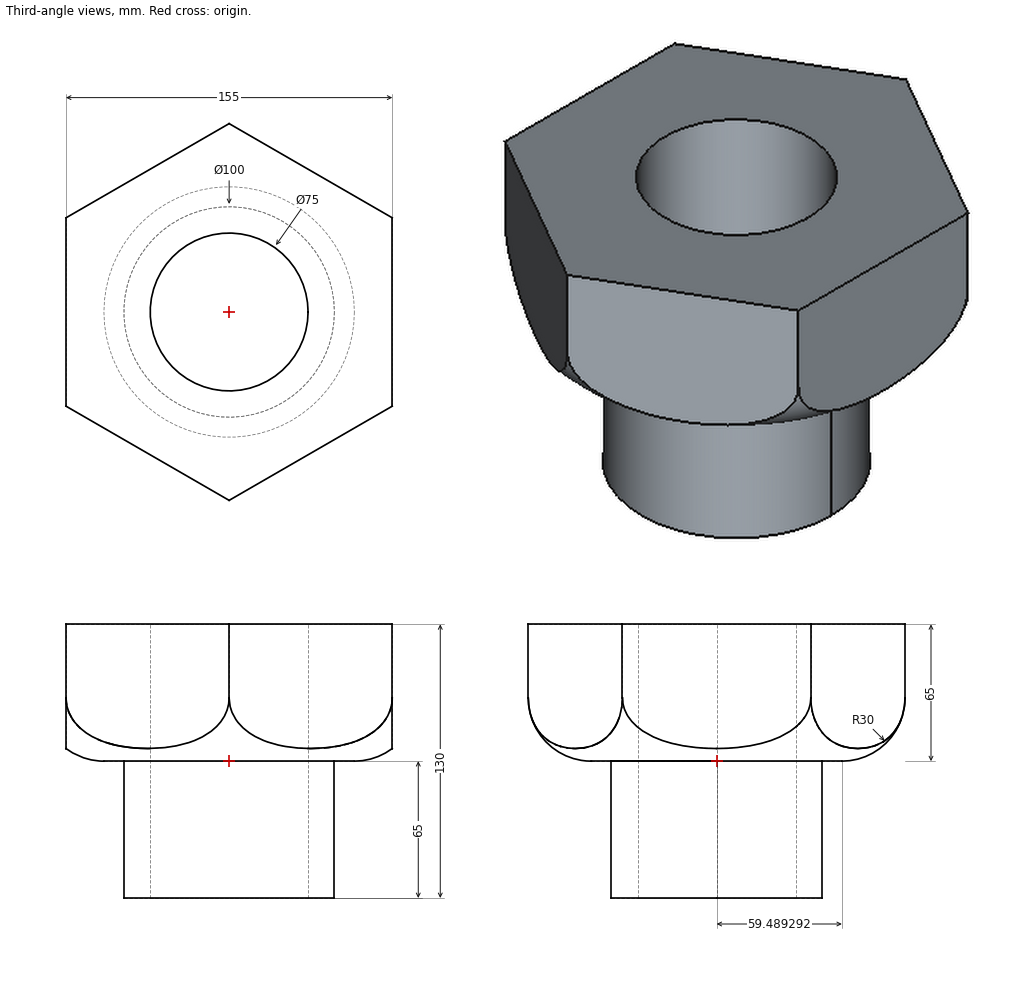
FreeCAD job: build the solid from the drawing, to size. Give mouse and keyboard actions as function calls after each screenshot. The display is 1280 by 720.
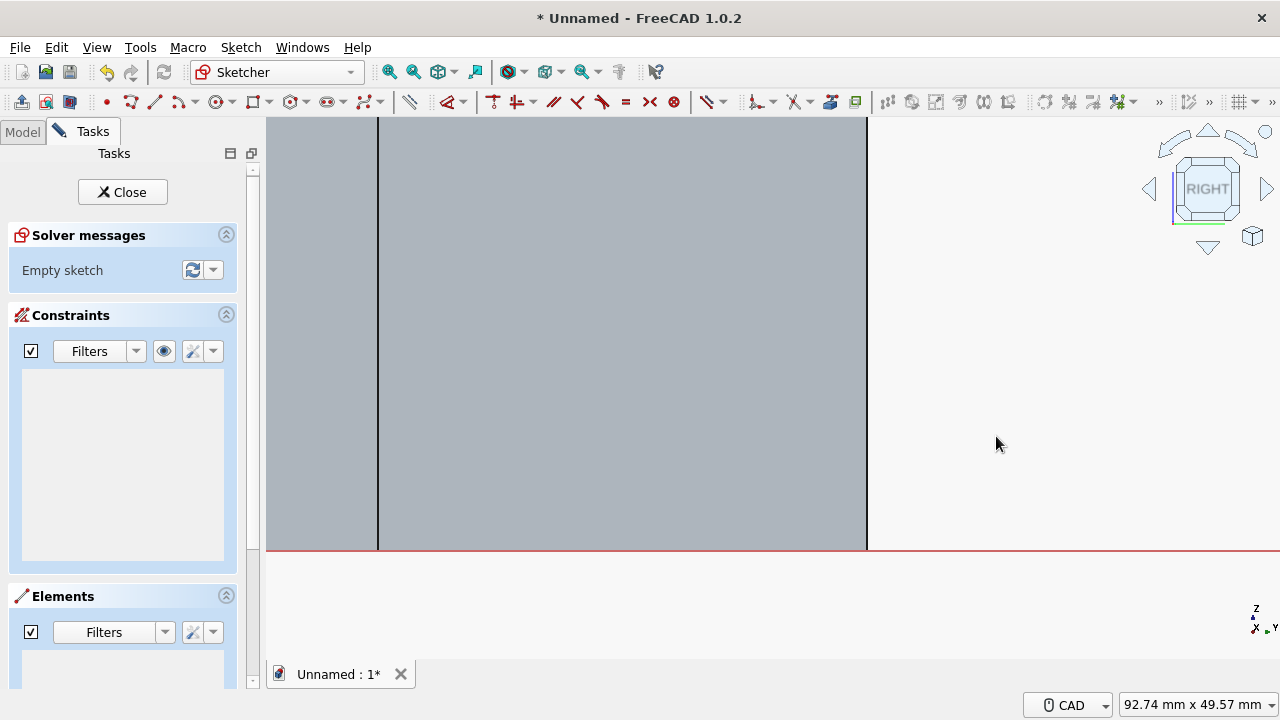
key(g)
key(m)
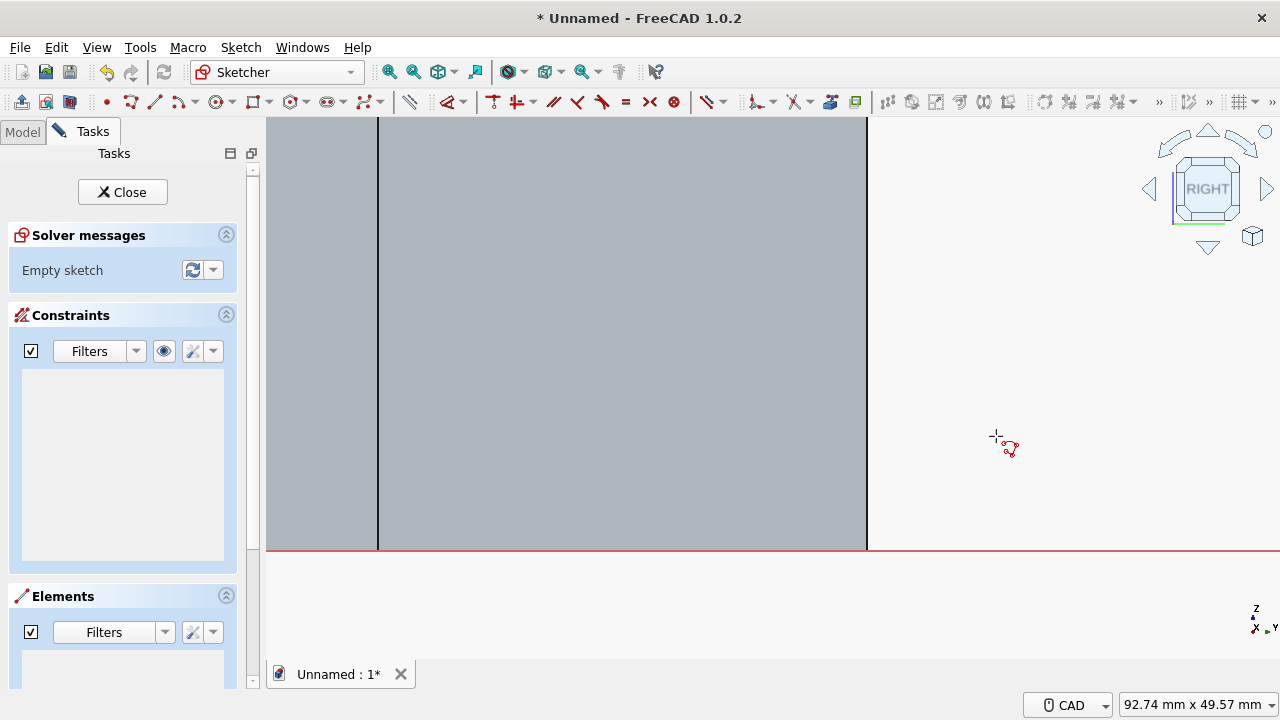
click(539, 551)
click(867, 542)
click(867, 223)
right_click(867, 223)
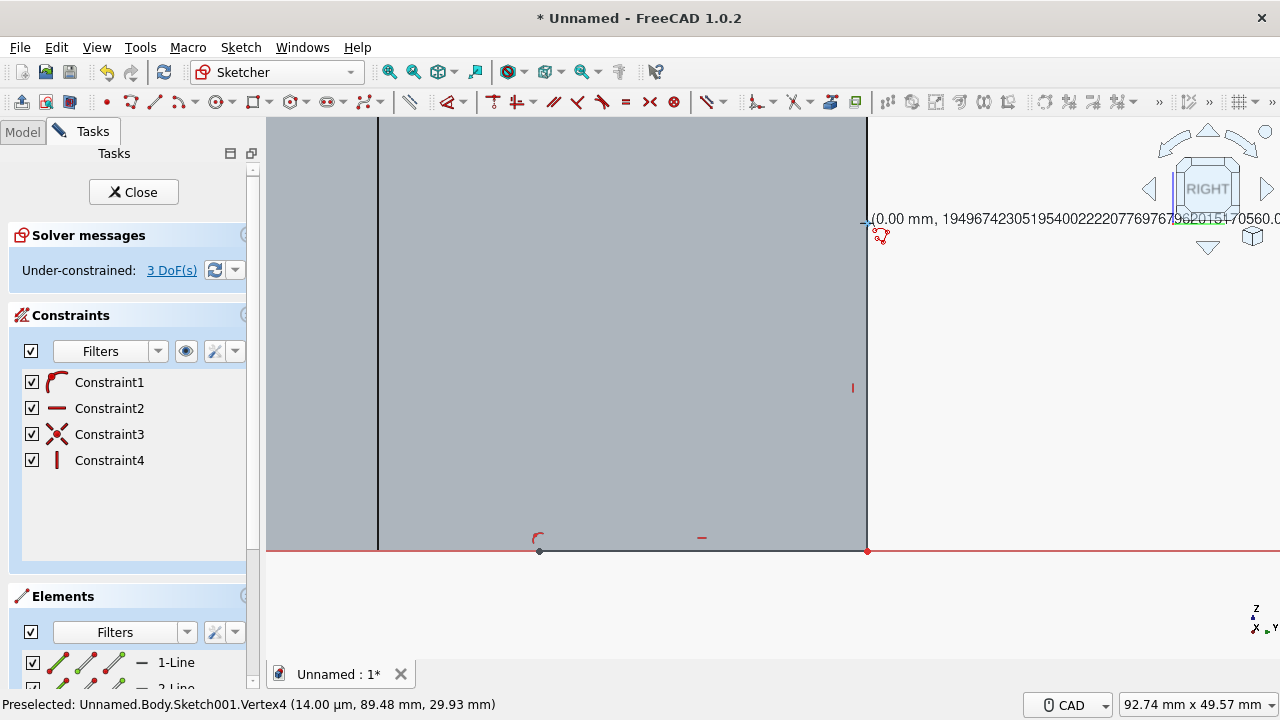
click(198, 102)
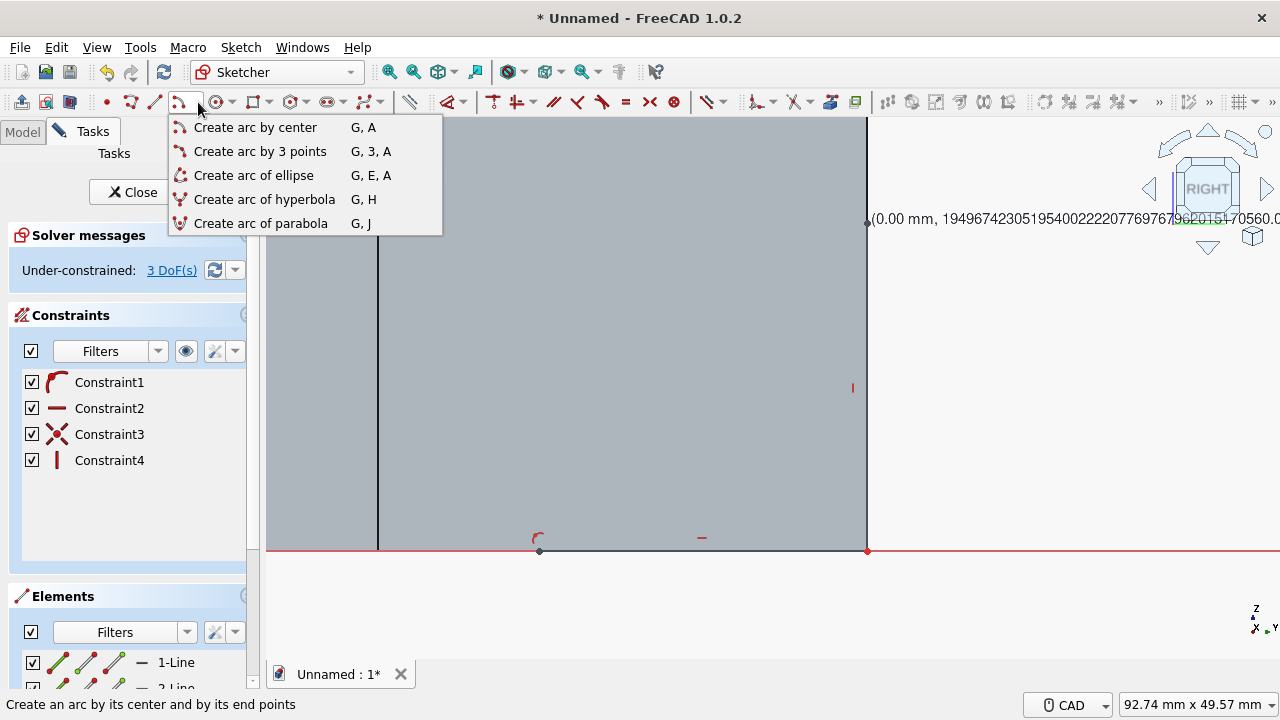
click(306, 151)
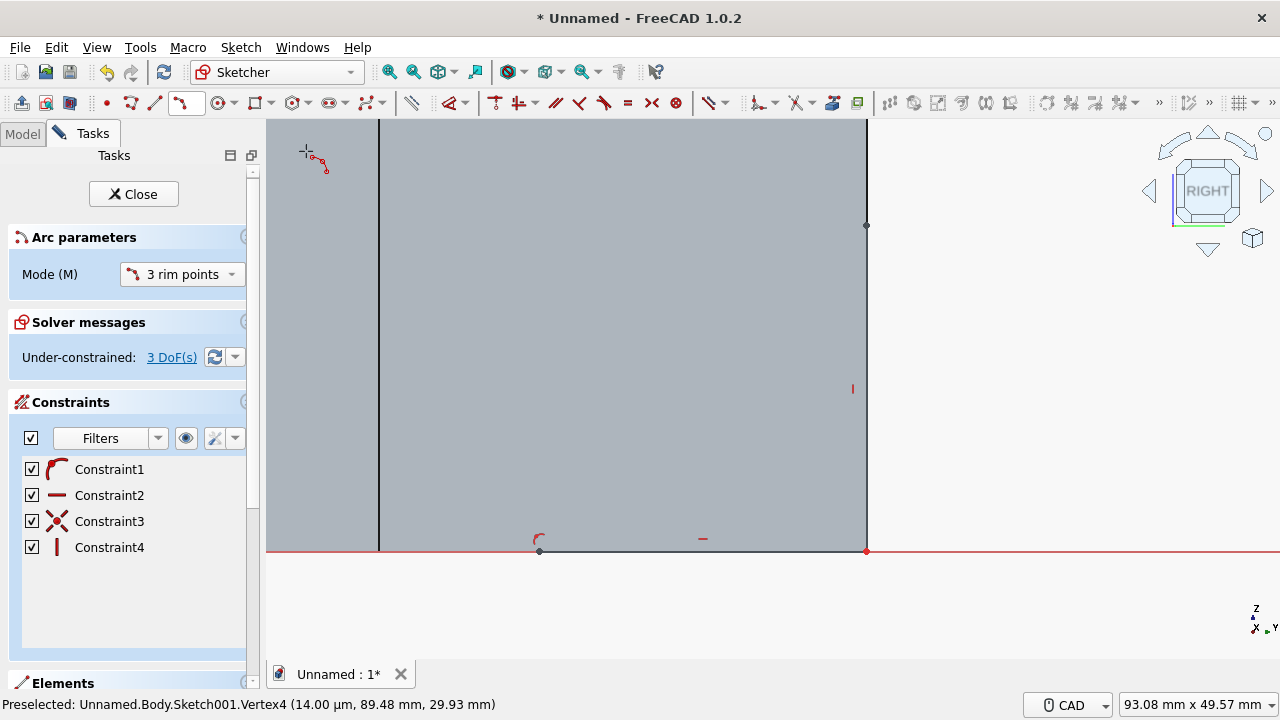
click(867, 226)
click(540, 552)
click(771, 456)
key(Escape)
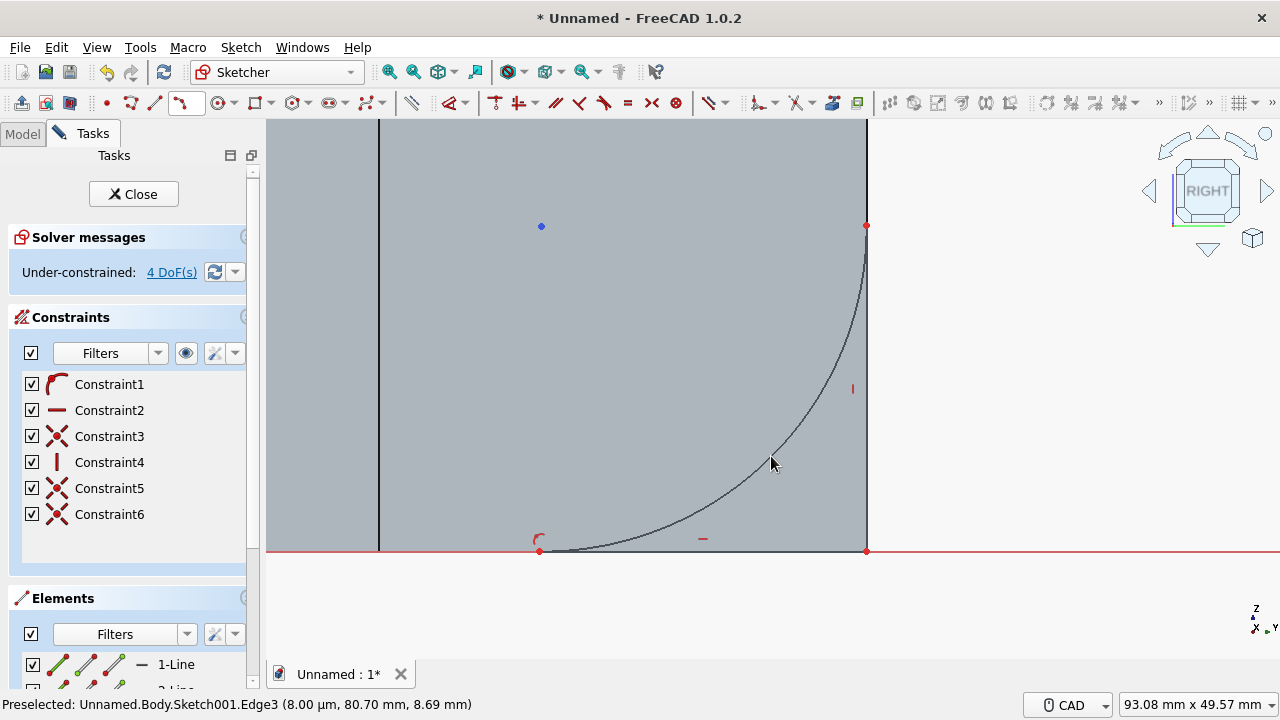
click(638, 552)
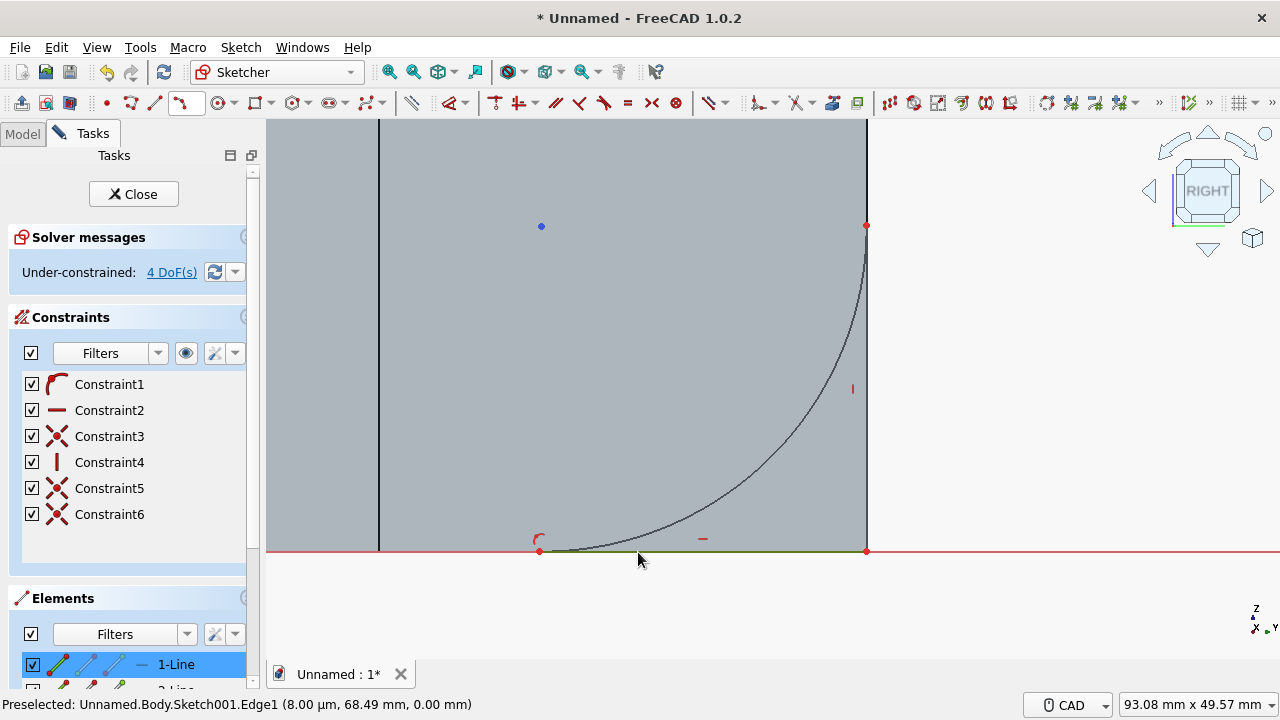
click(688, 517)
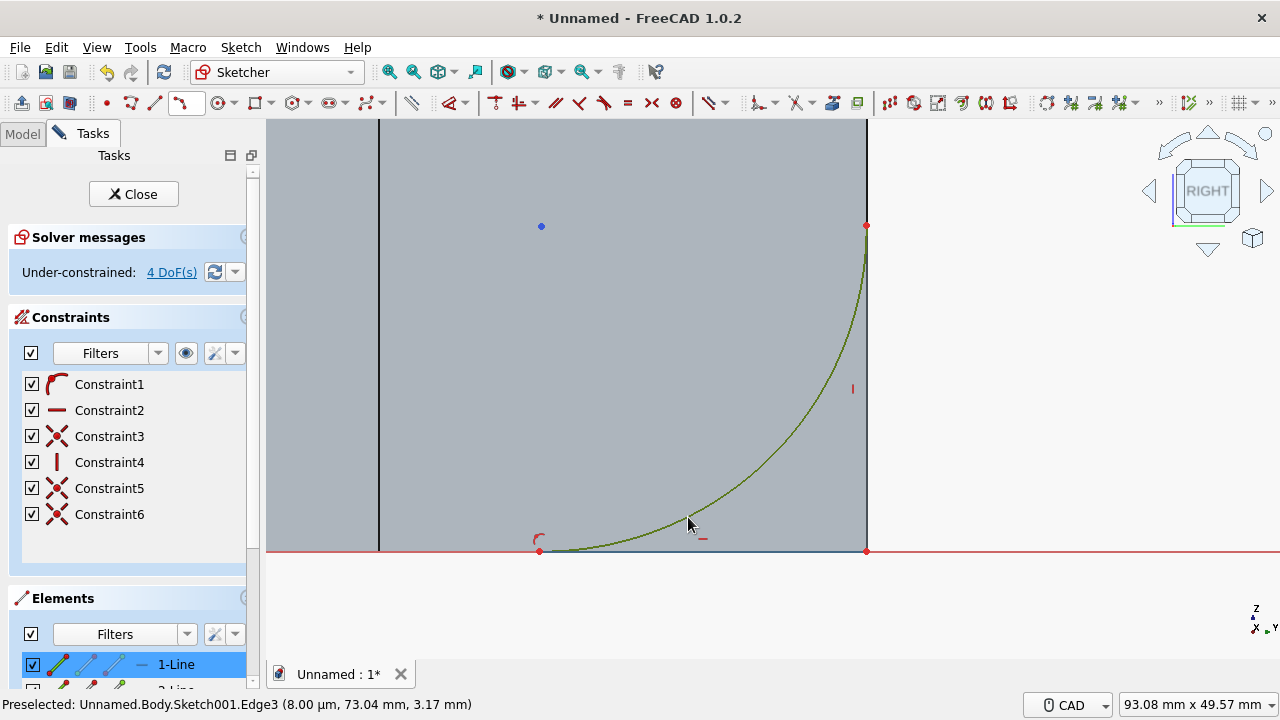
key(t)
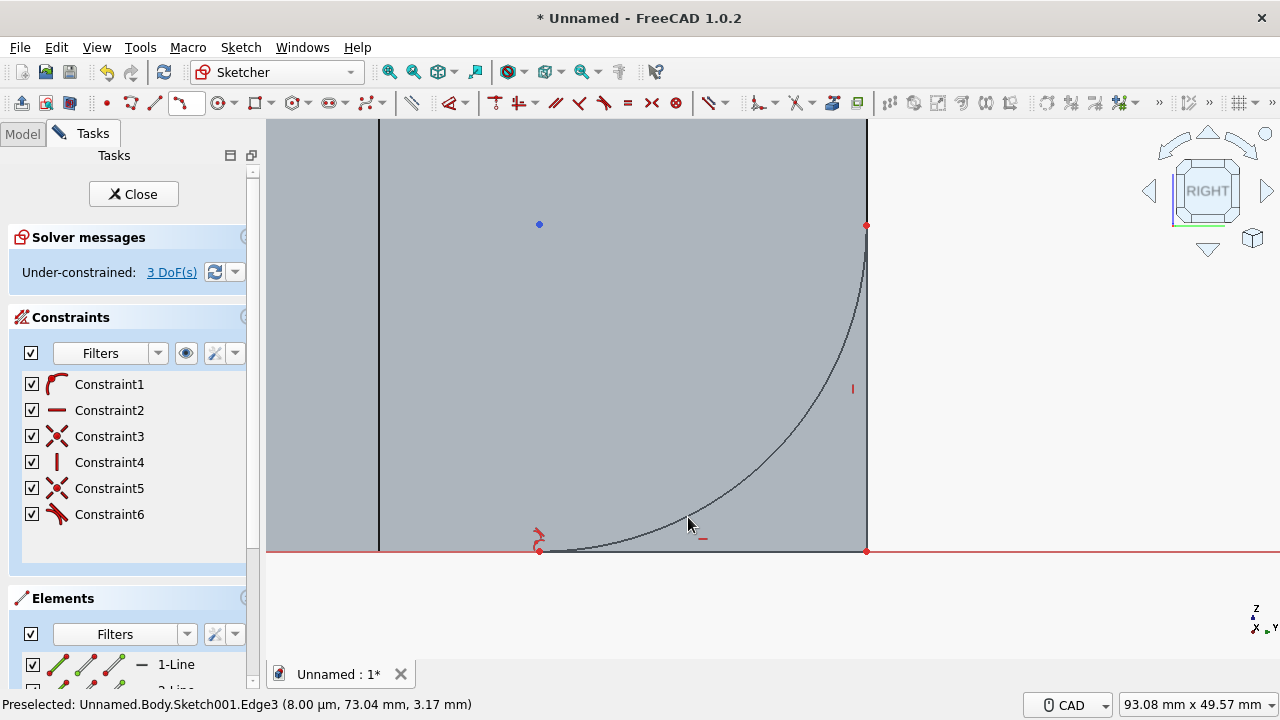
click(867, 454)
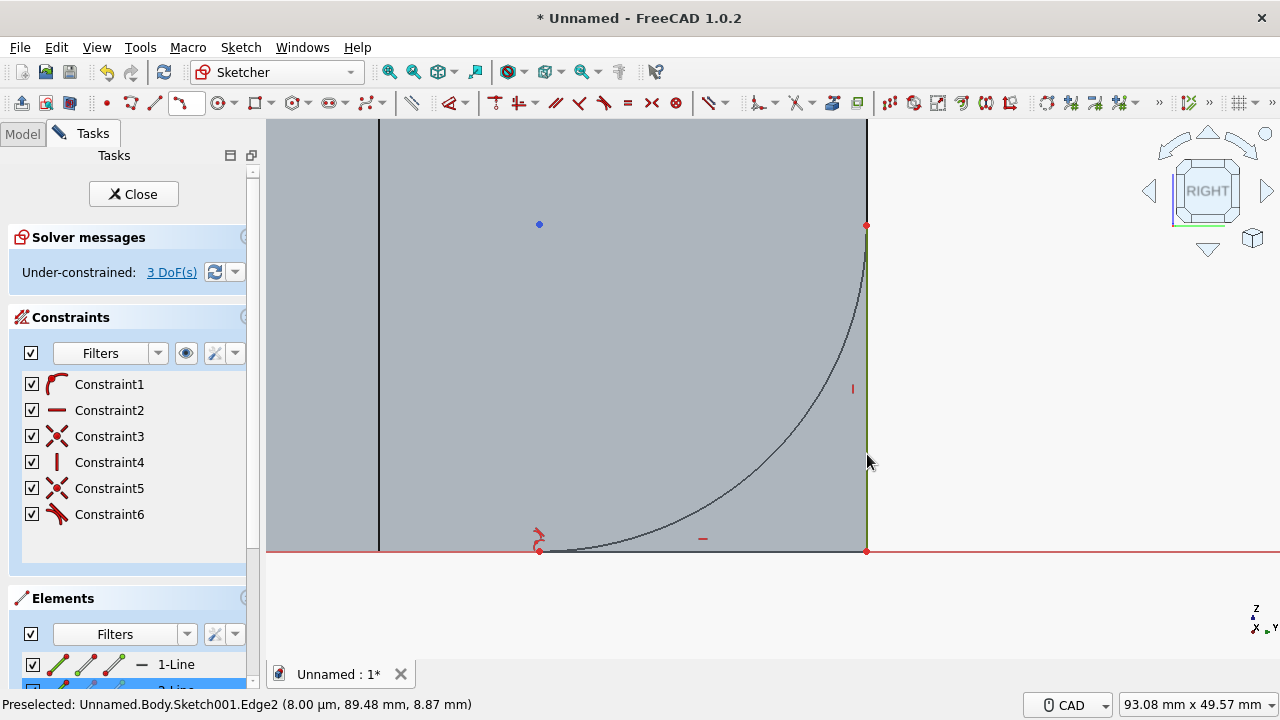
click(688, 516)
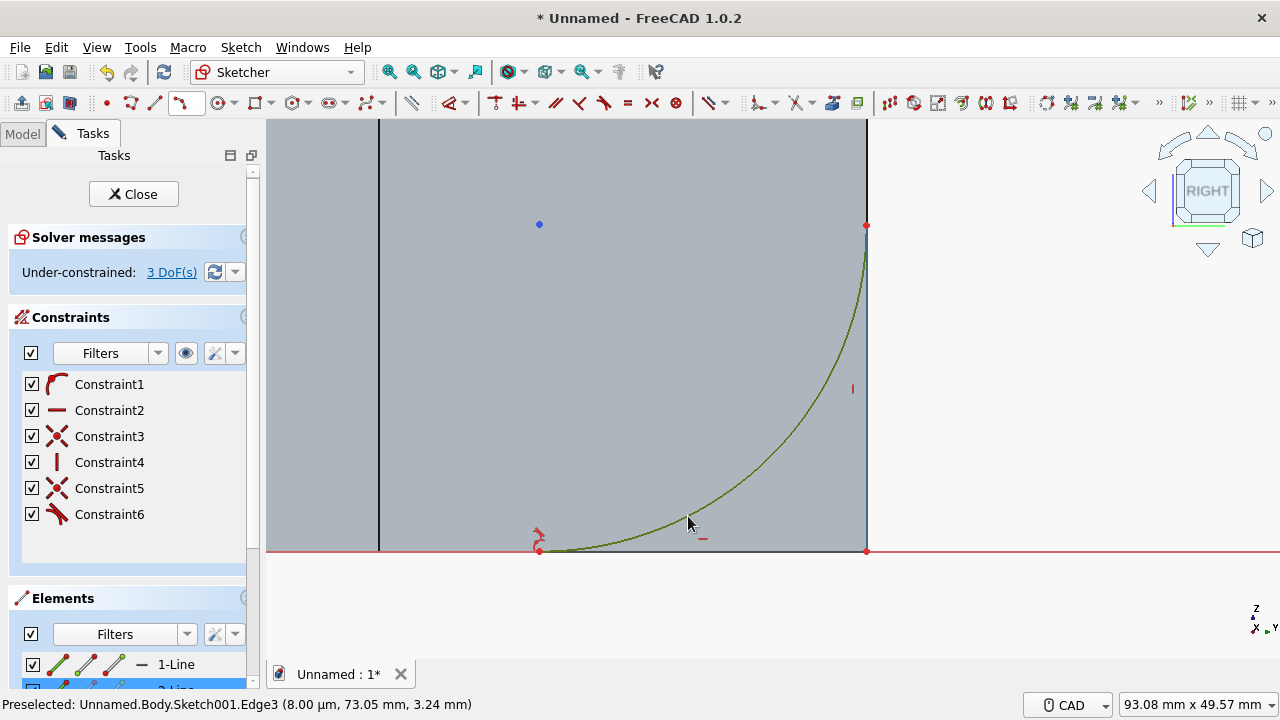
click(604, 104)